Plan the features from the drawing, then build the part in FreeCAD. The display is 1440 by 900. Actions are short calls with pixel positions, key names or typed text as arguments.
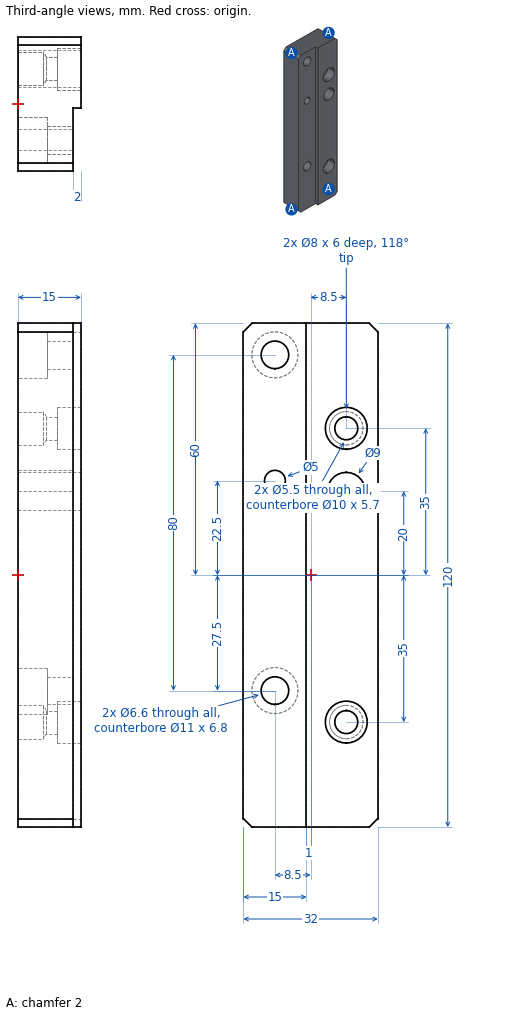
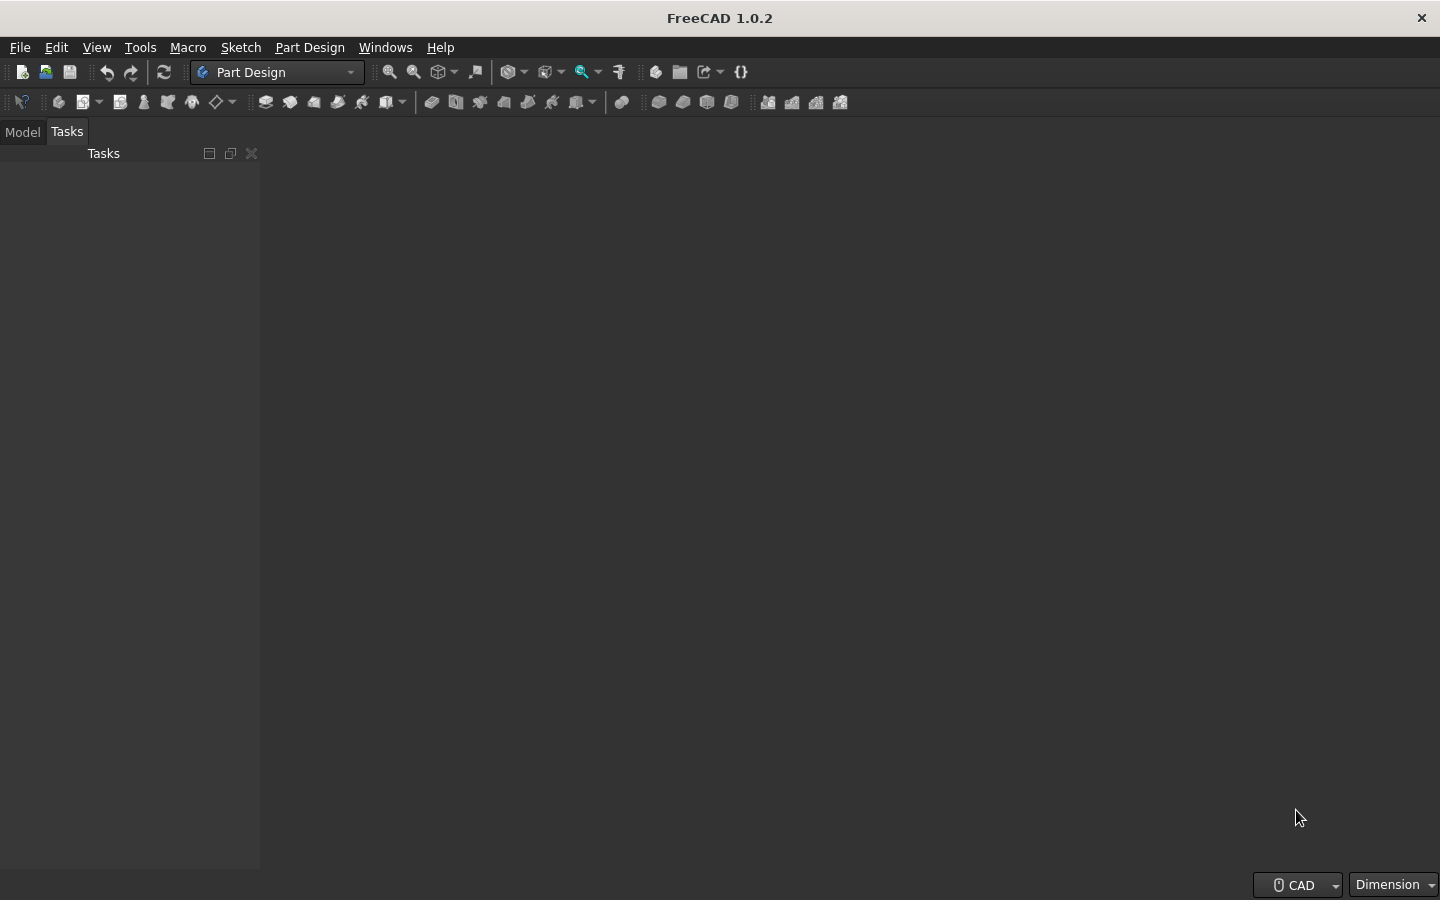
click(248, 72)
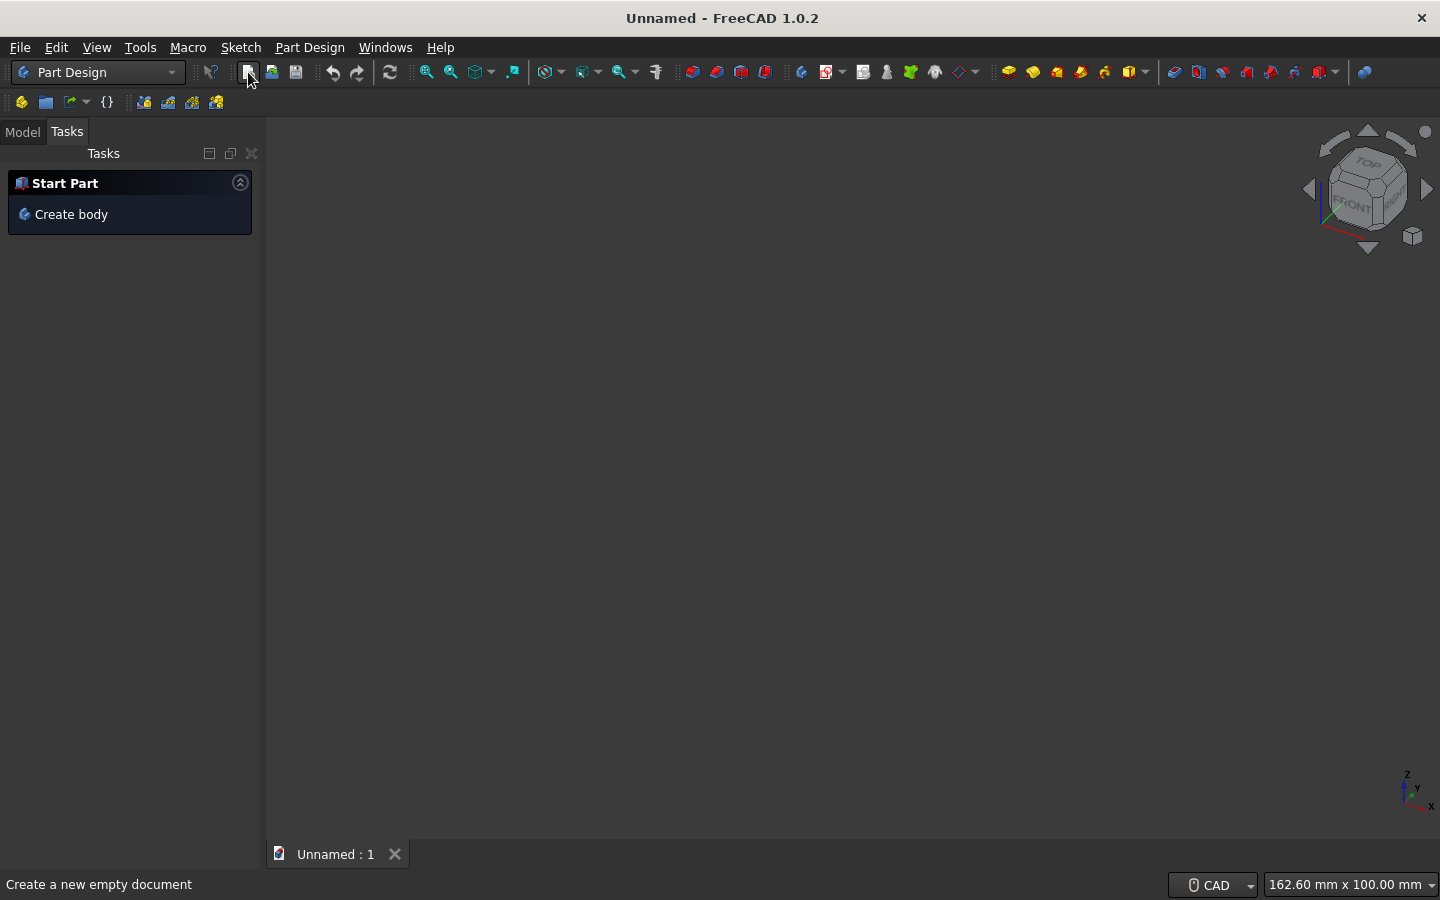
click(826, 72)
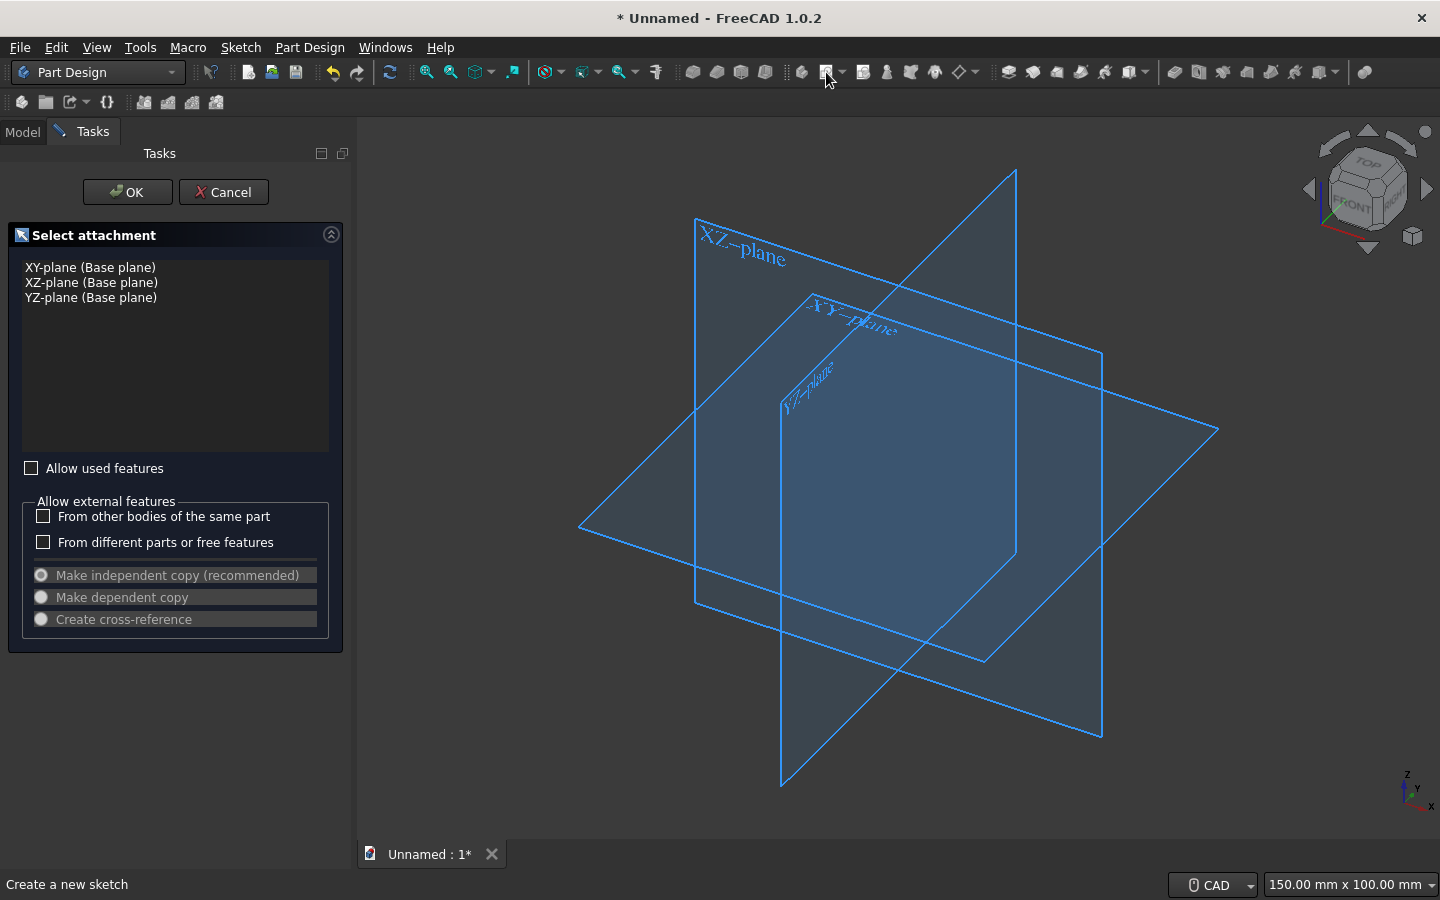
click(82, 298)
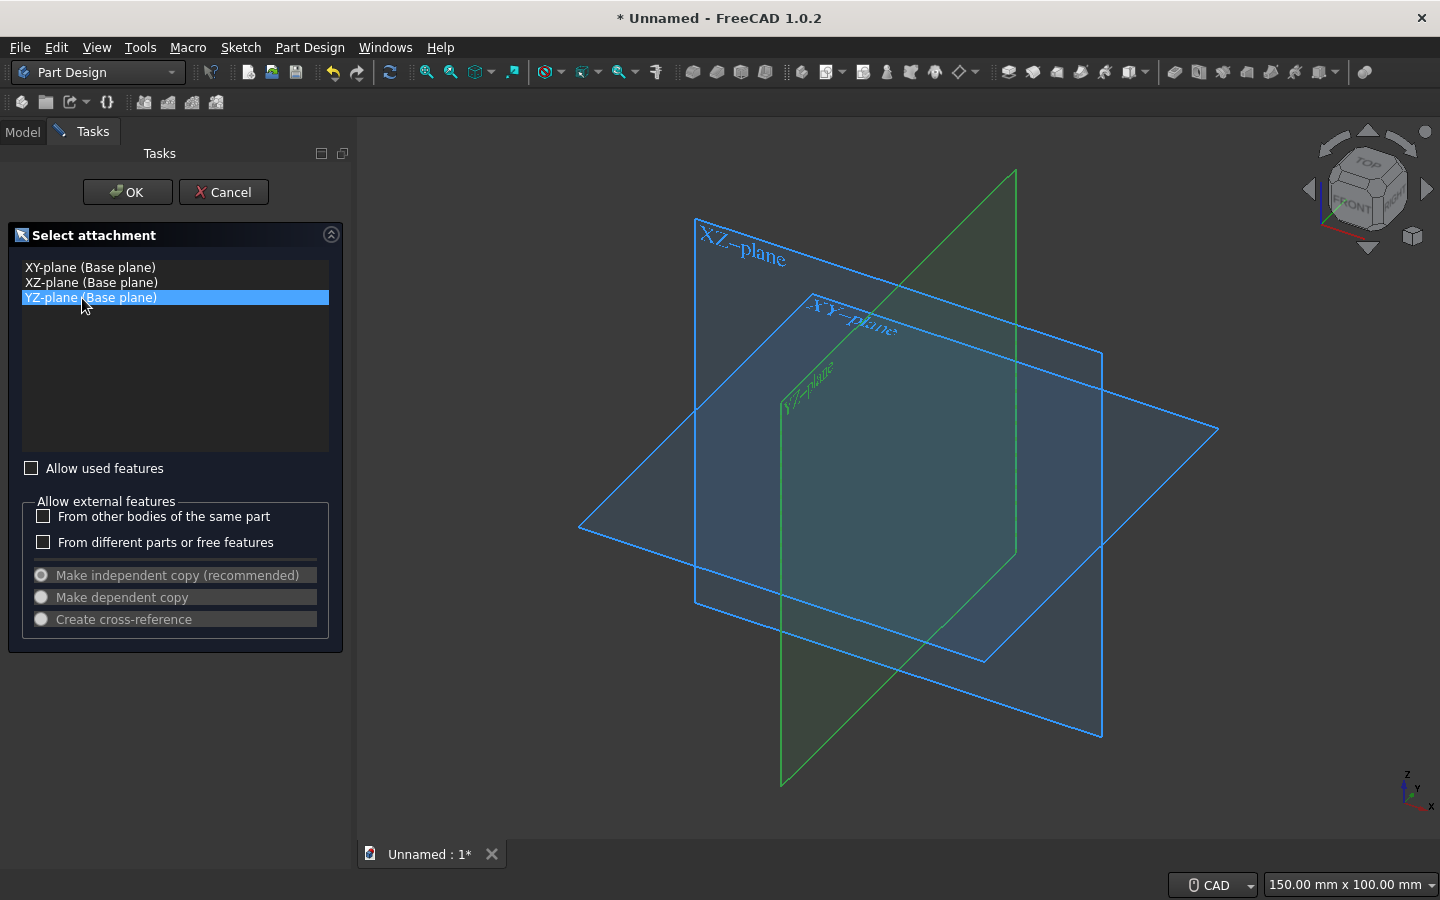
click(128, 192)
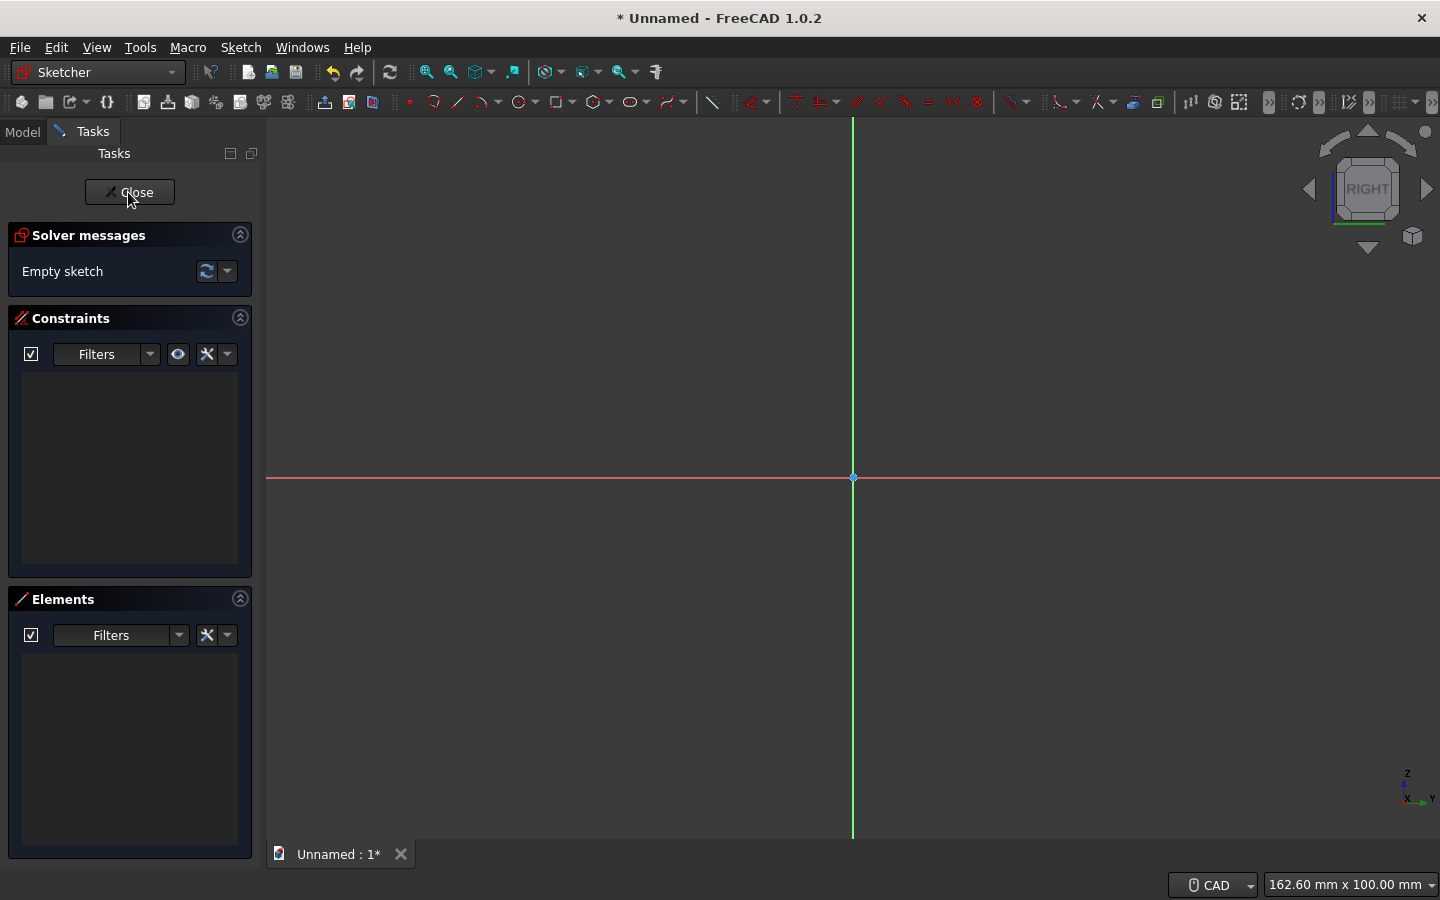
scroll(701, 478, down, 3)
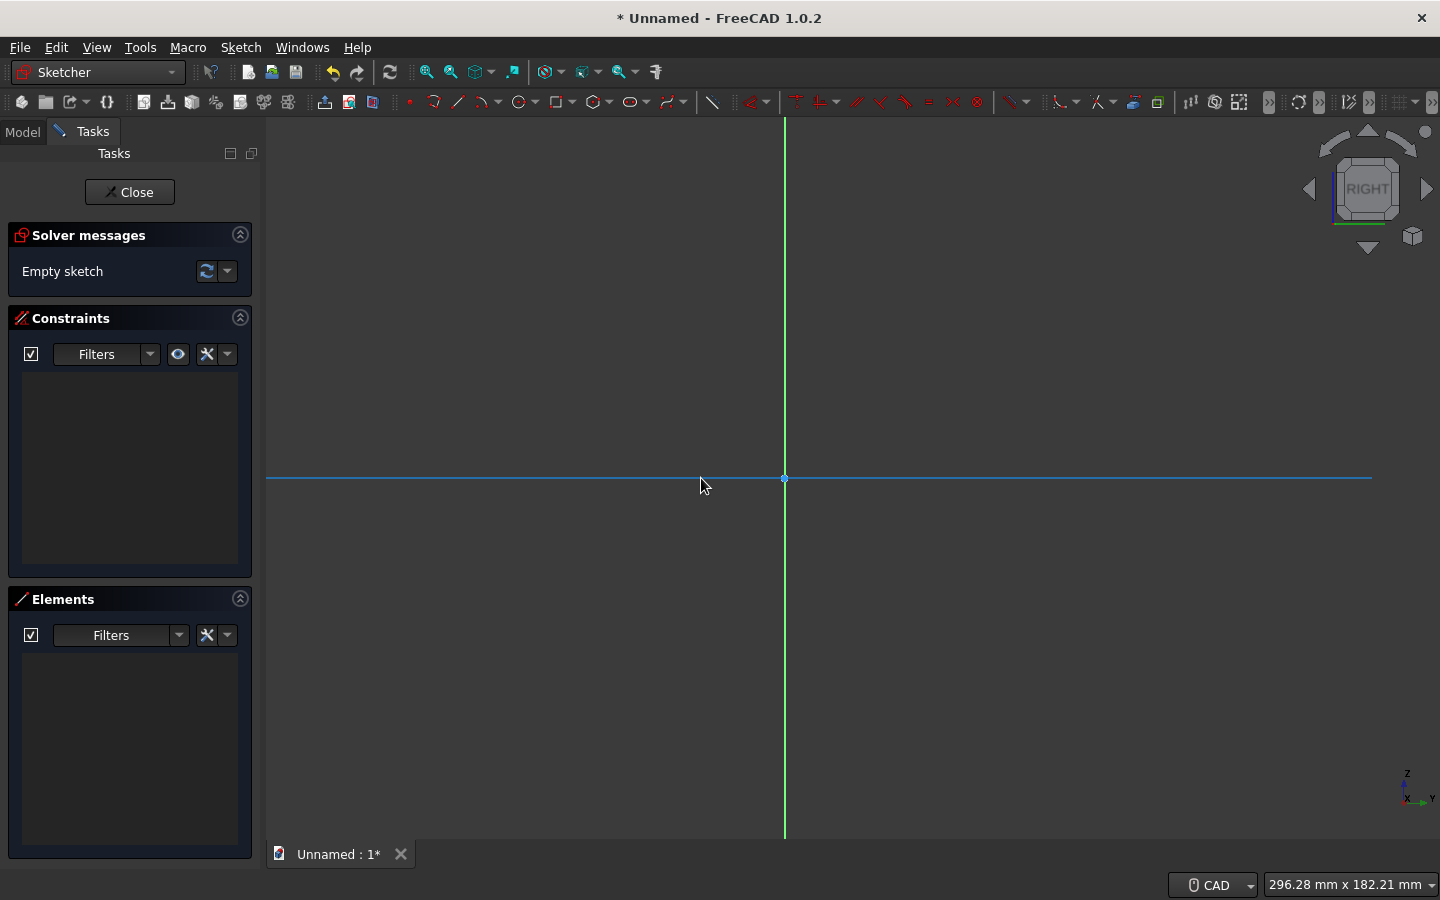
key(g)
key(v)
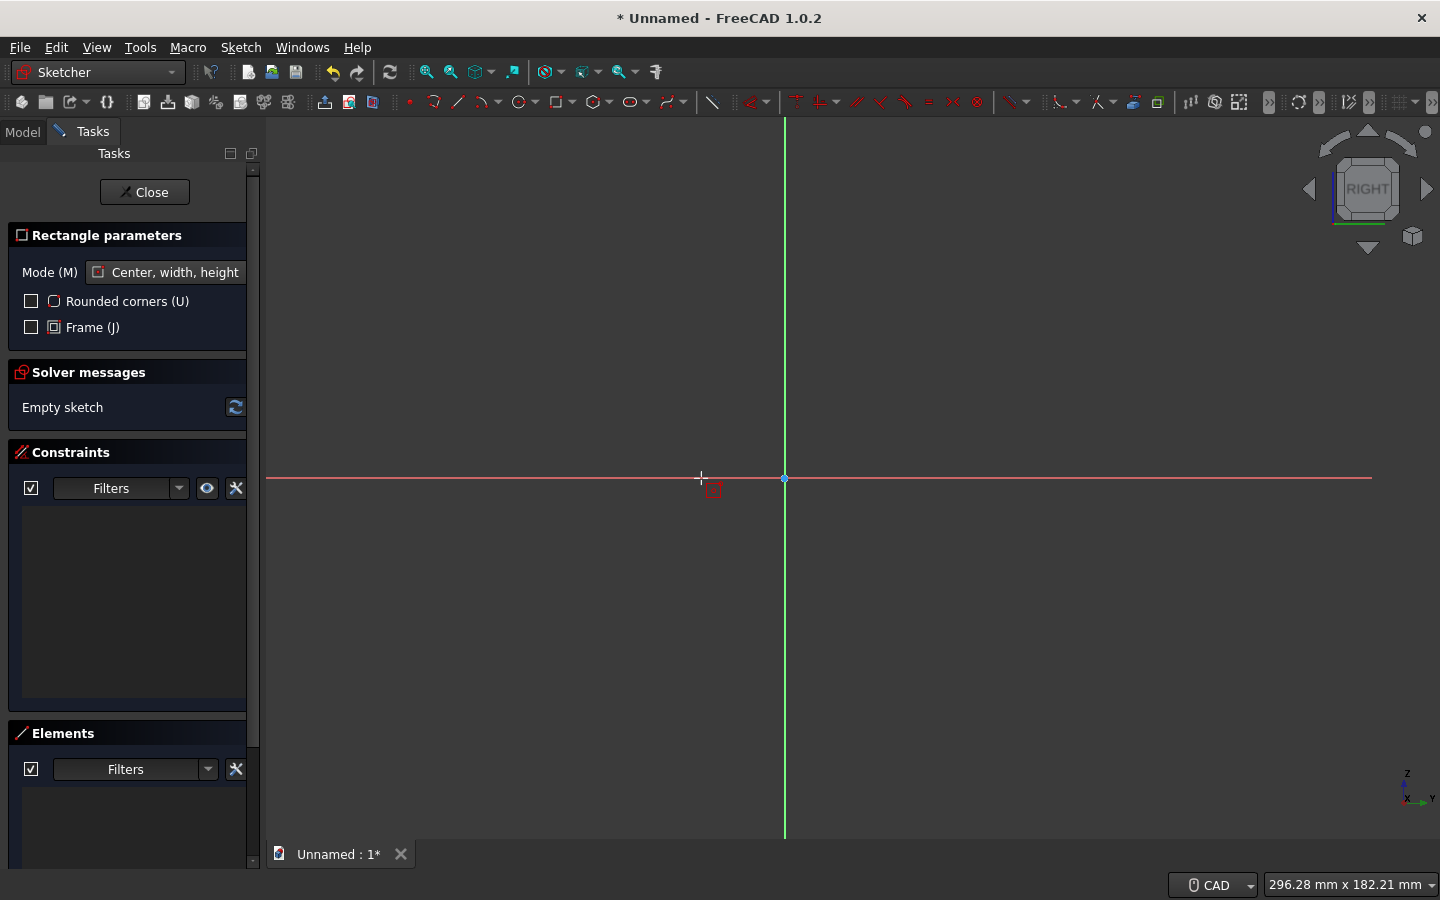
click(785, 478)
click(848, 240)
key(Escape)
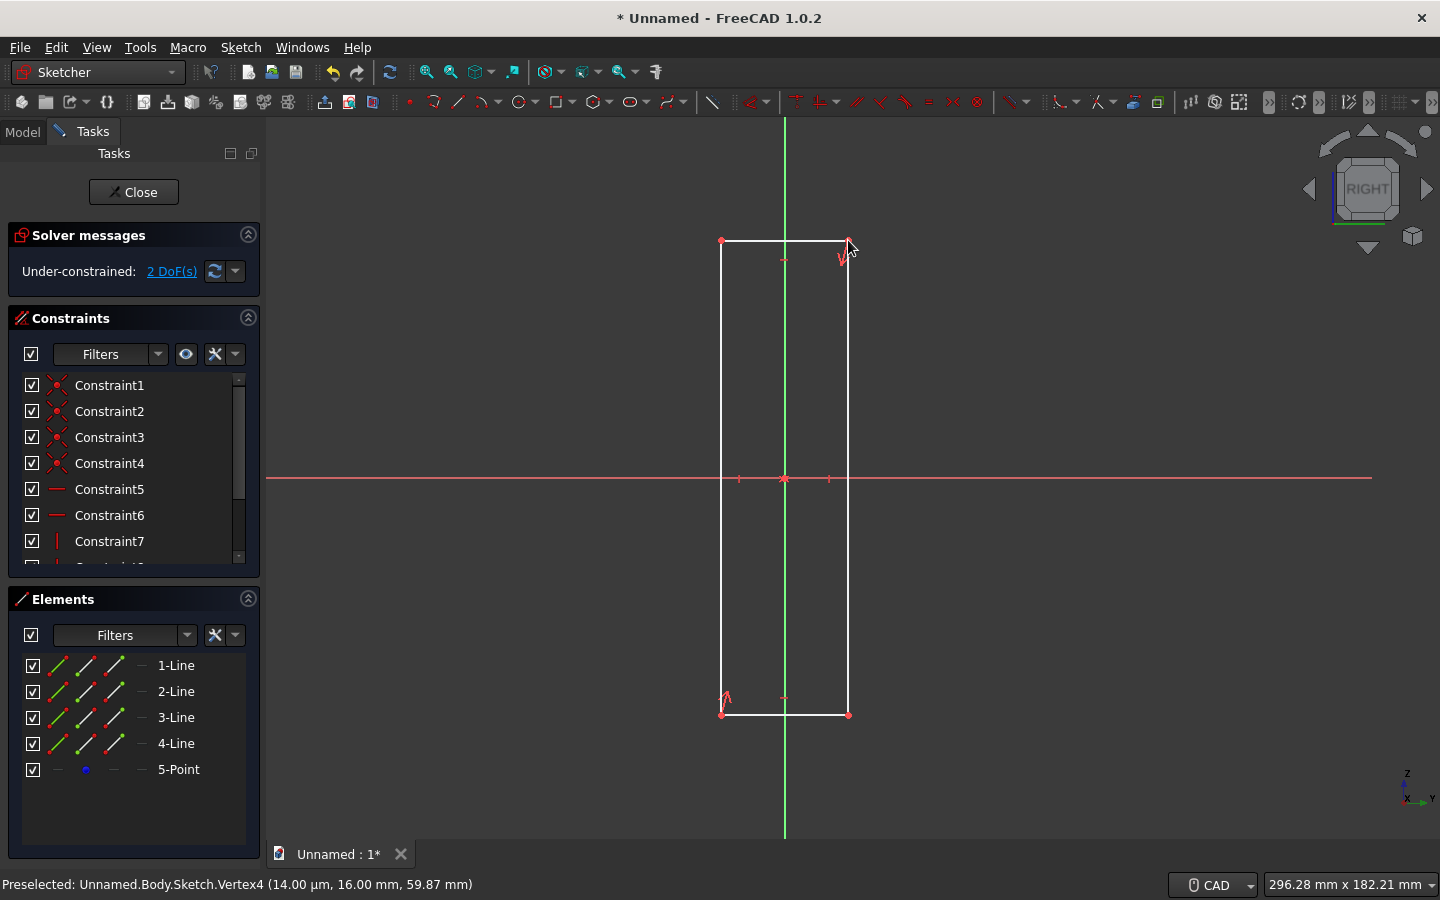
click(750, 102)